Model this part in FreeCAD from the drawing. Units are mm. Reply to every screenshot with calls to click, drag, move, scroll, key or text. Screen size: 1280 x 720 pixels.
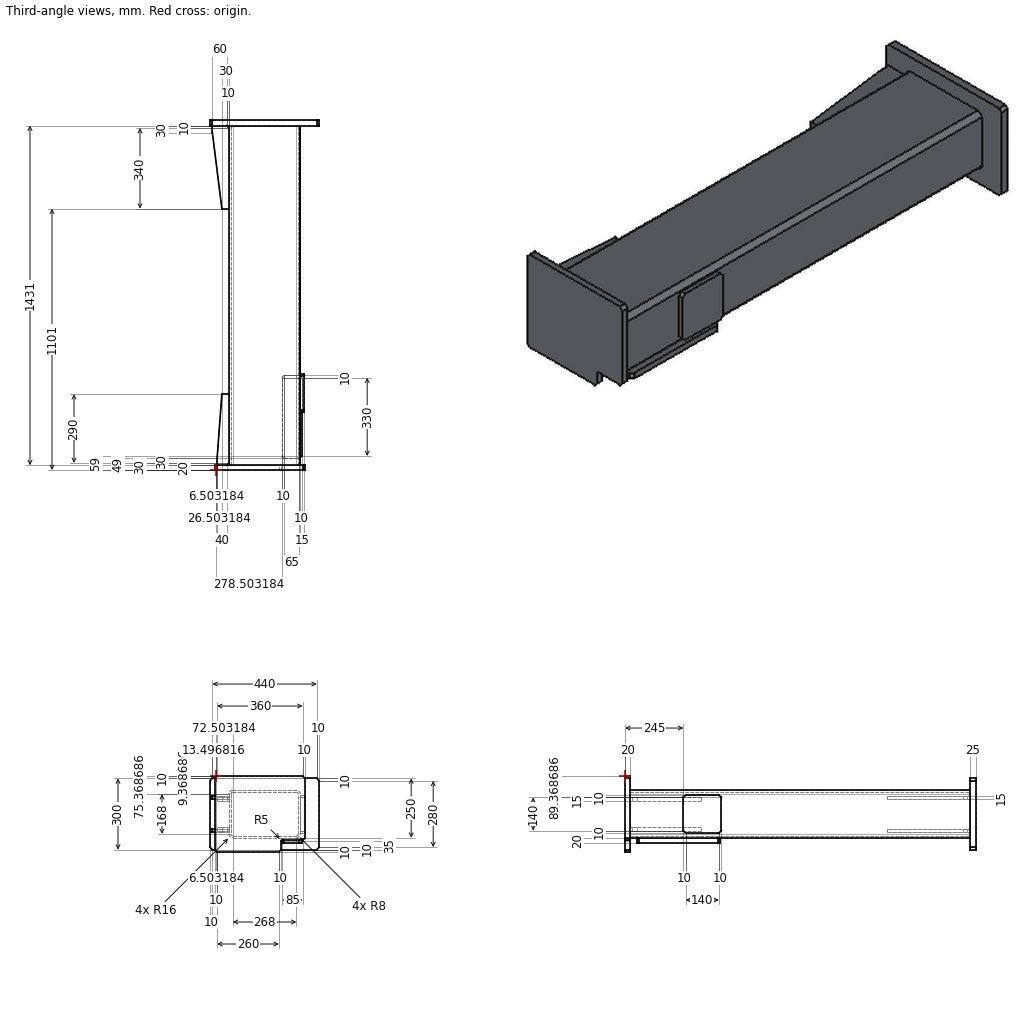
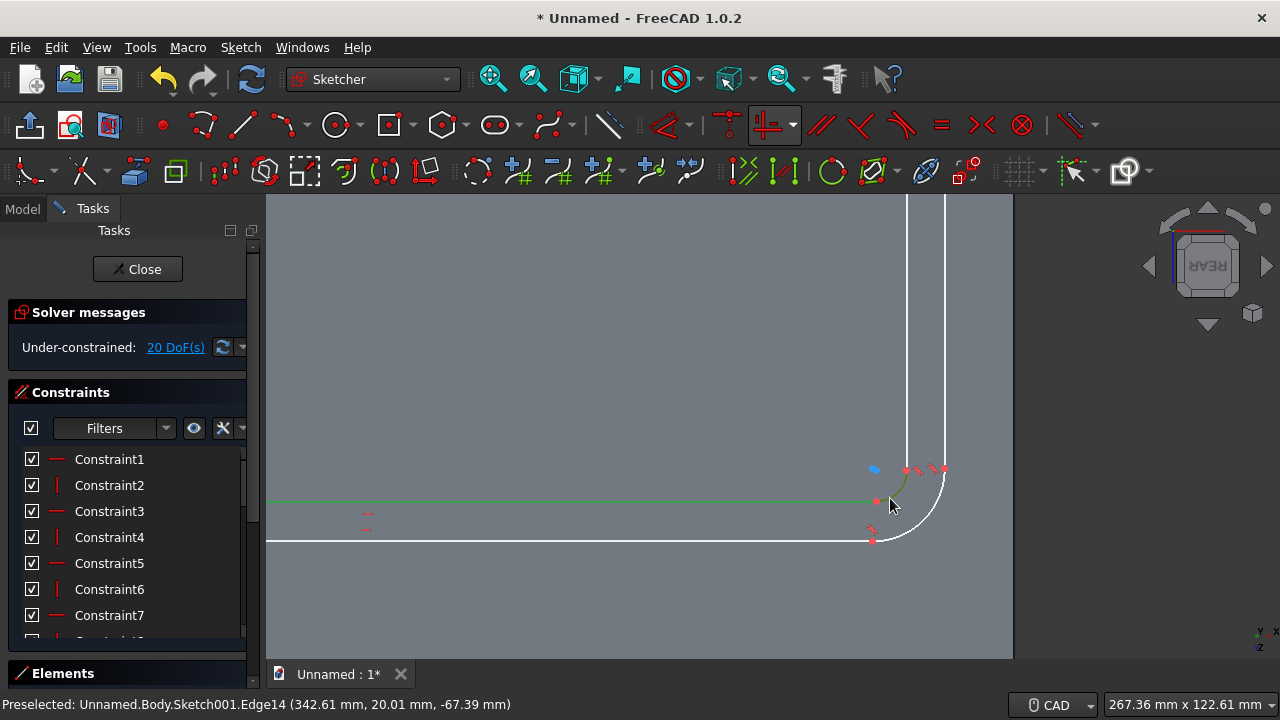
click(902, 126)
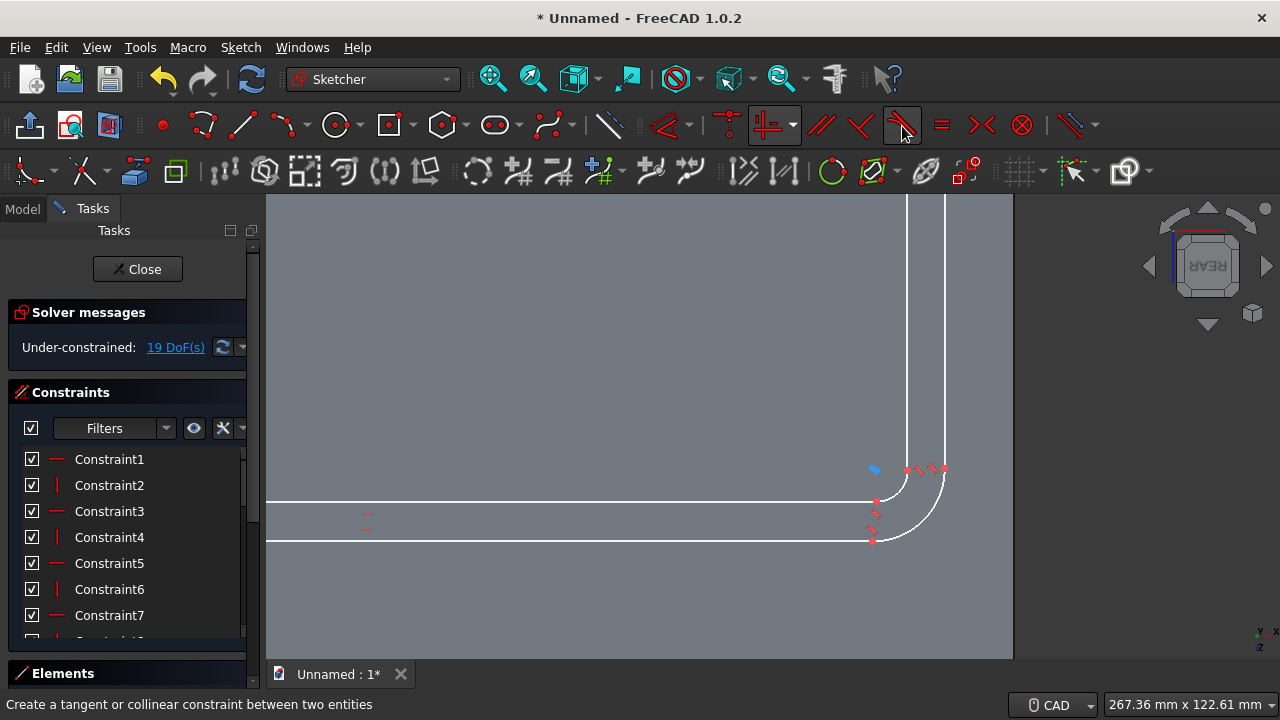
scroll(895, 497, down, 6)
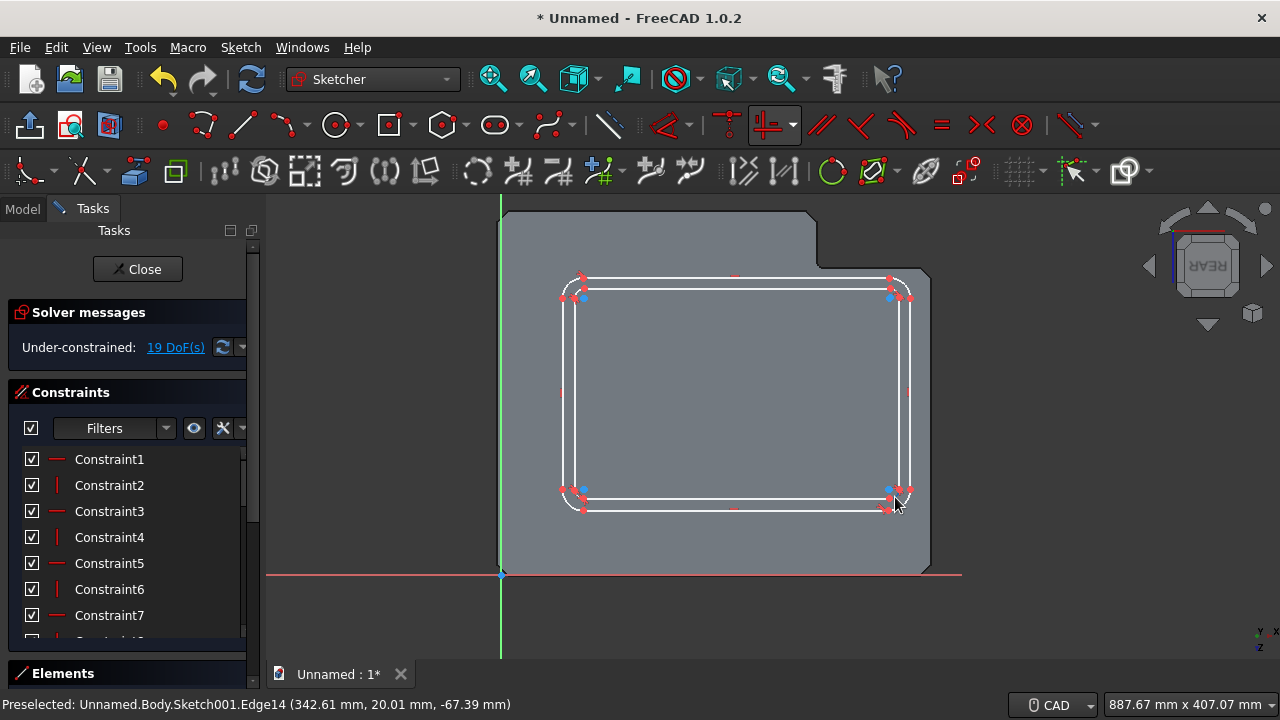
click(798, 499)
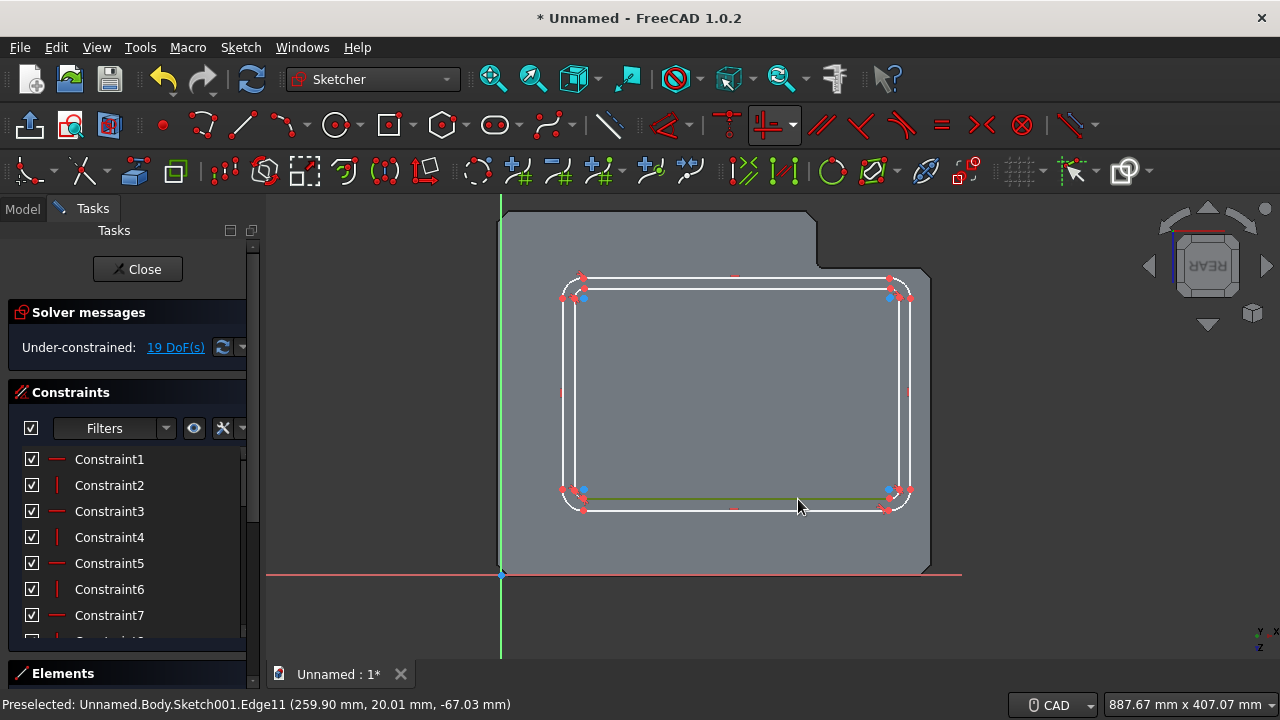
scroll(578, 496, up, 4)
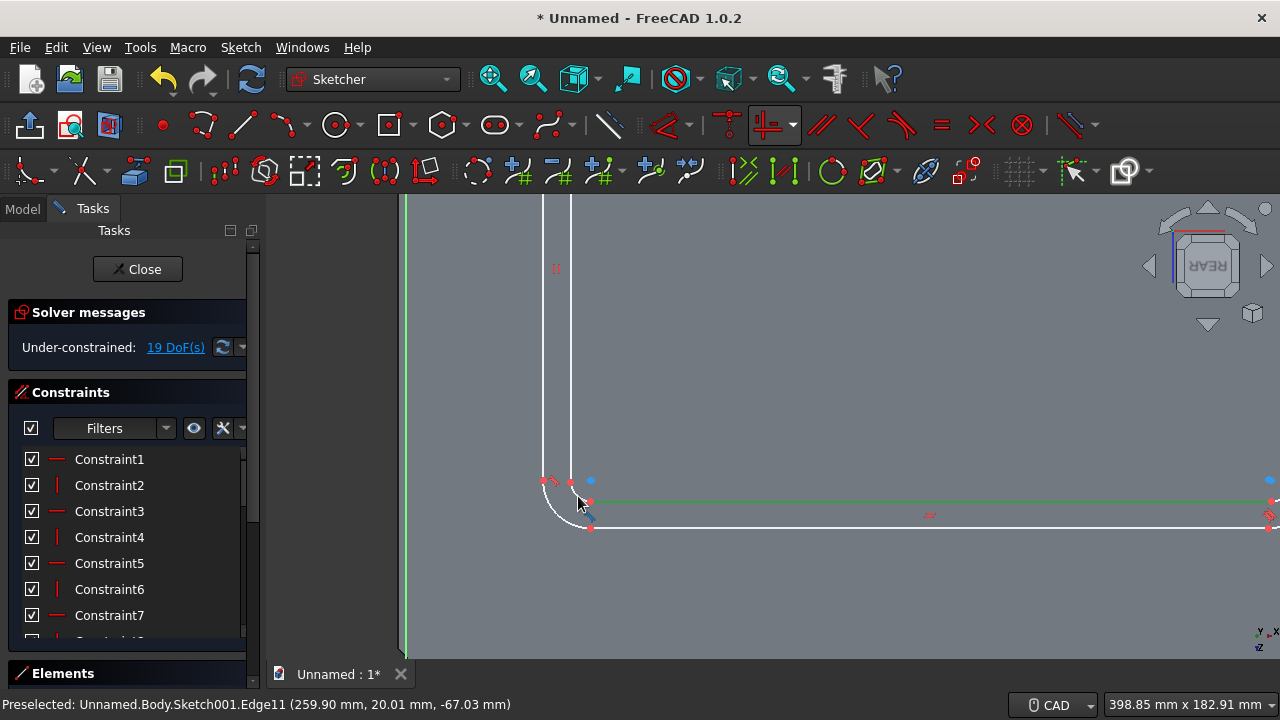
click(577, 495)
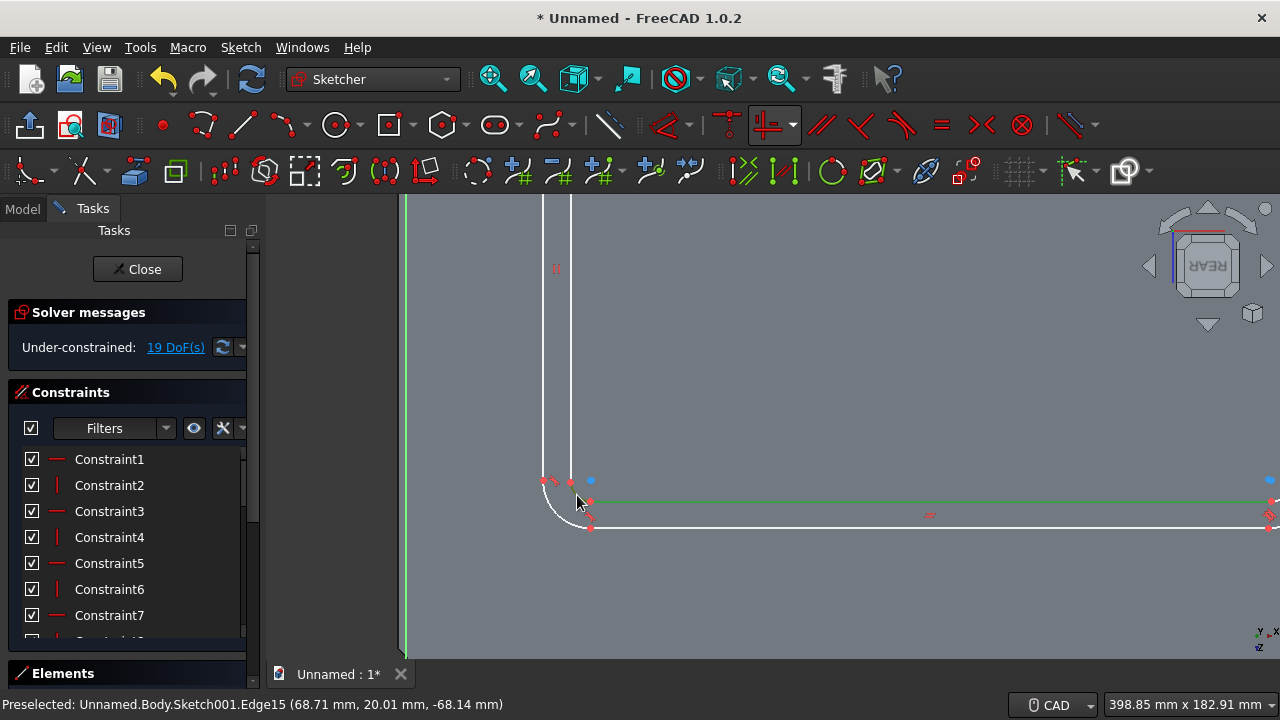
click(902, 126)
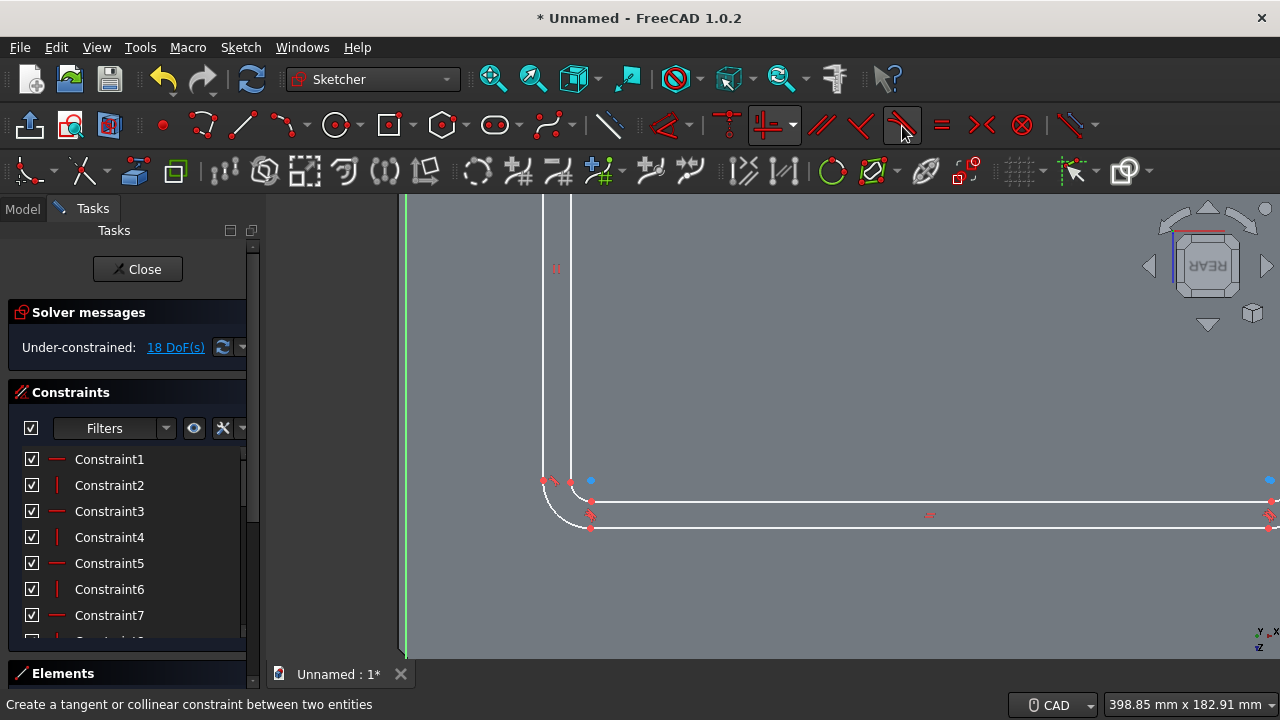
click(571, 354)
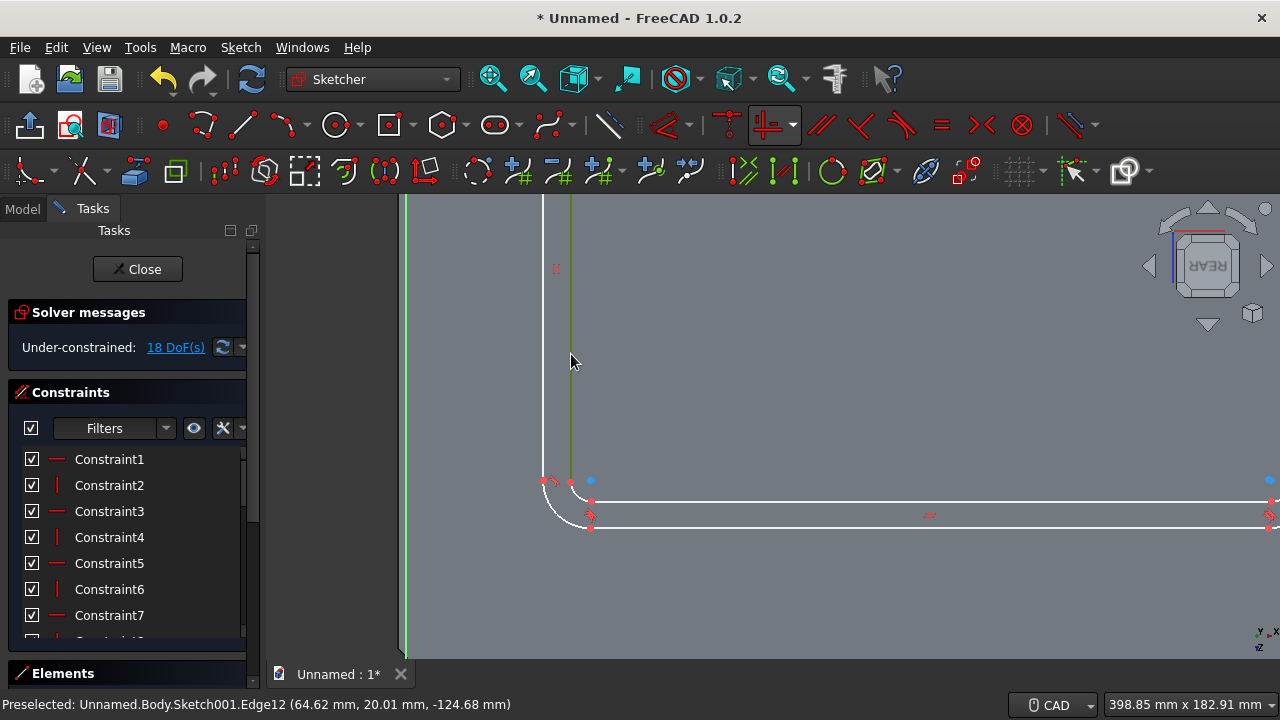
scroll(574, 491, up, 2)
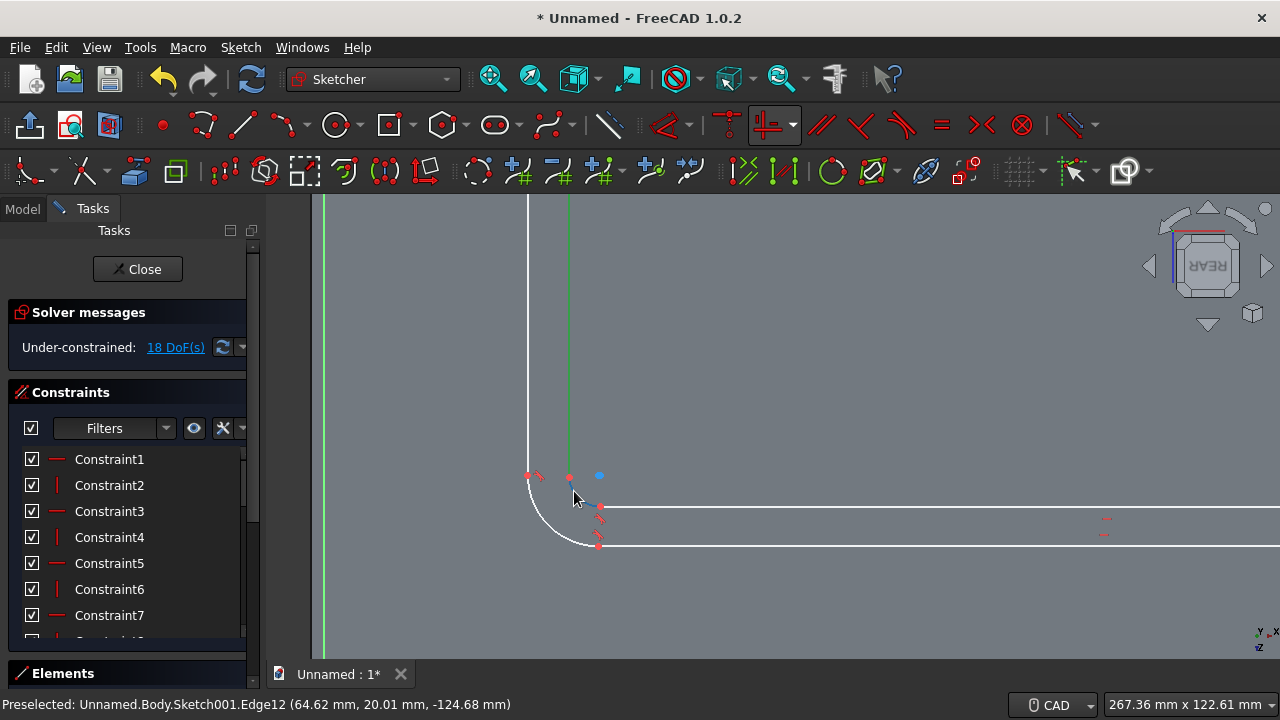
click(573, 491)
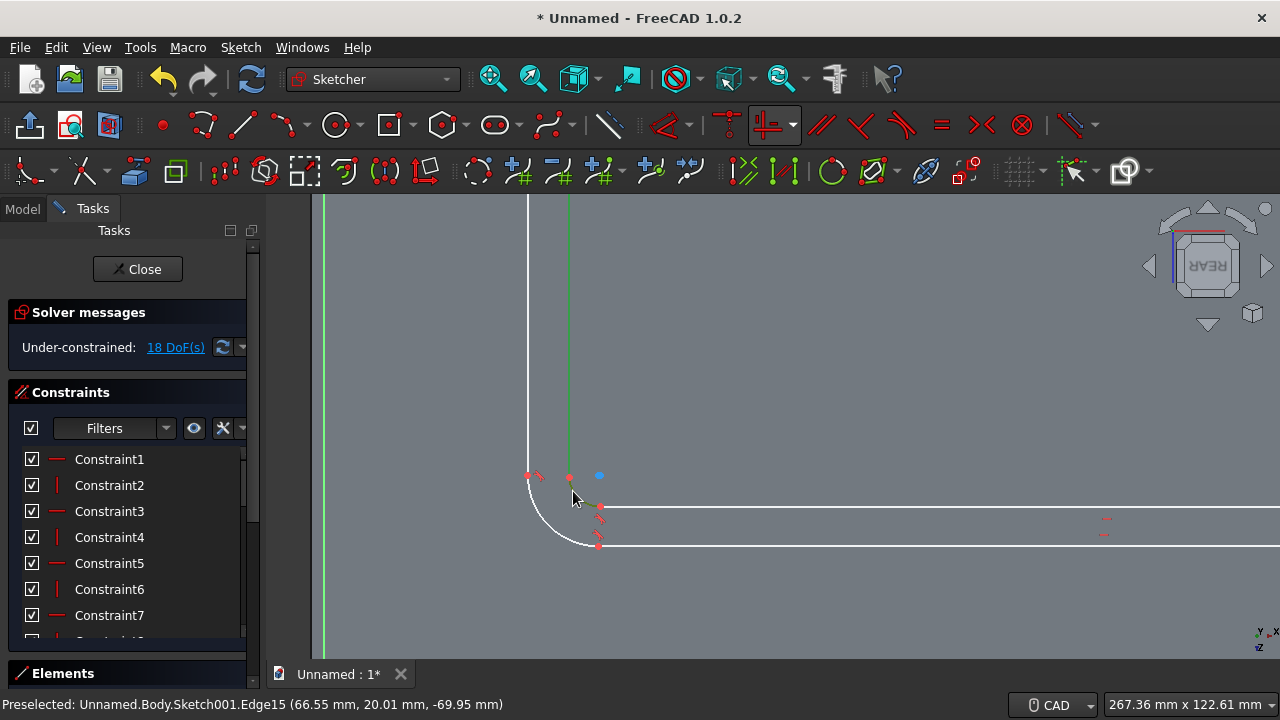
click(902, 126)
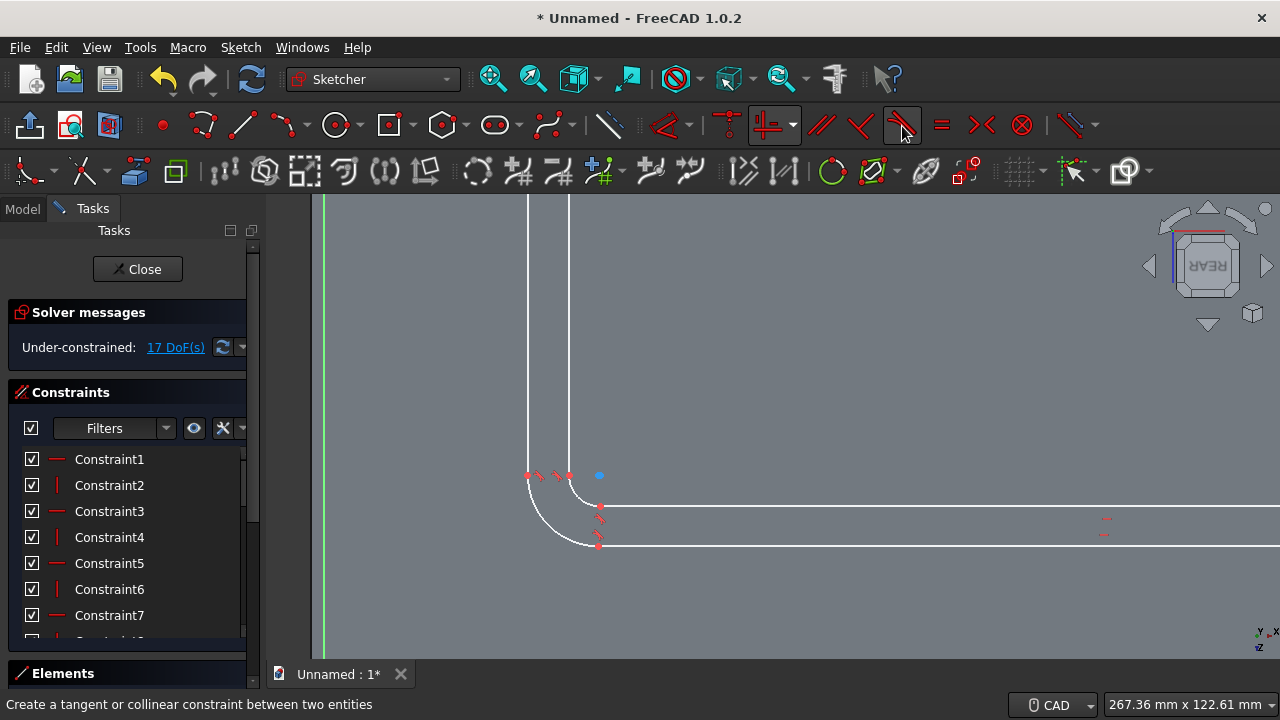
scroll(577, 494, down, 6)